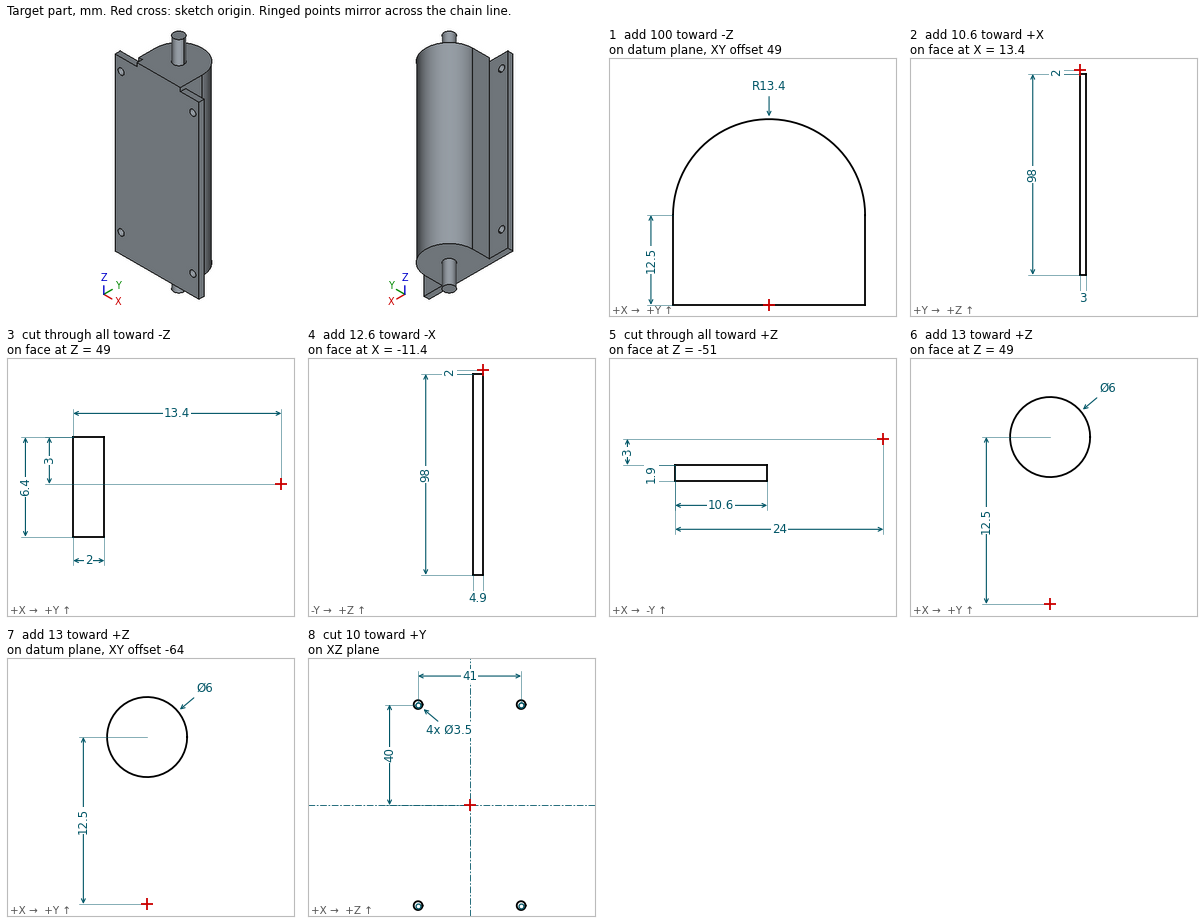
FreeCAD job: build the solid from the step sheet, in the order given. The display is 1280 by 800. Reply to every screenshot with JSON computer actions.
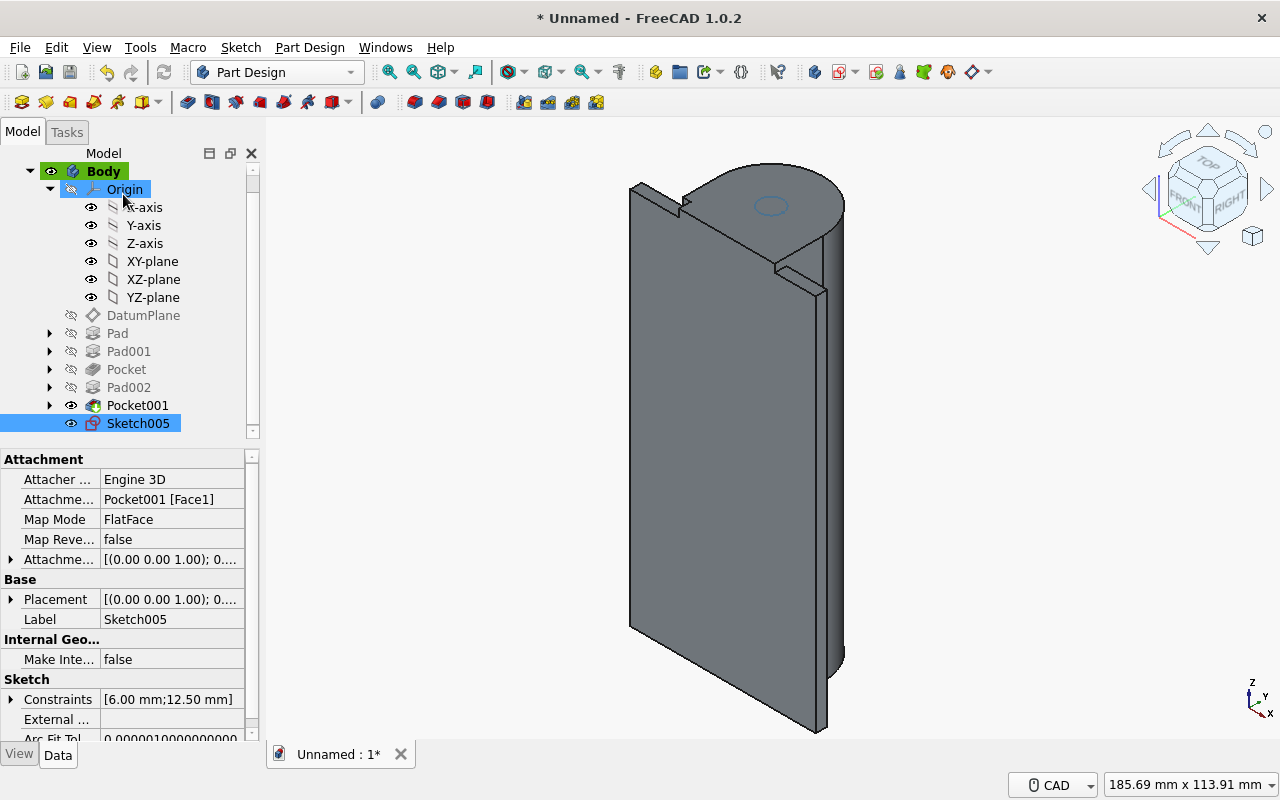
{"action": "left_click", "coordinate": [22, 102]}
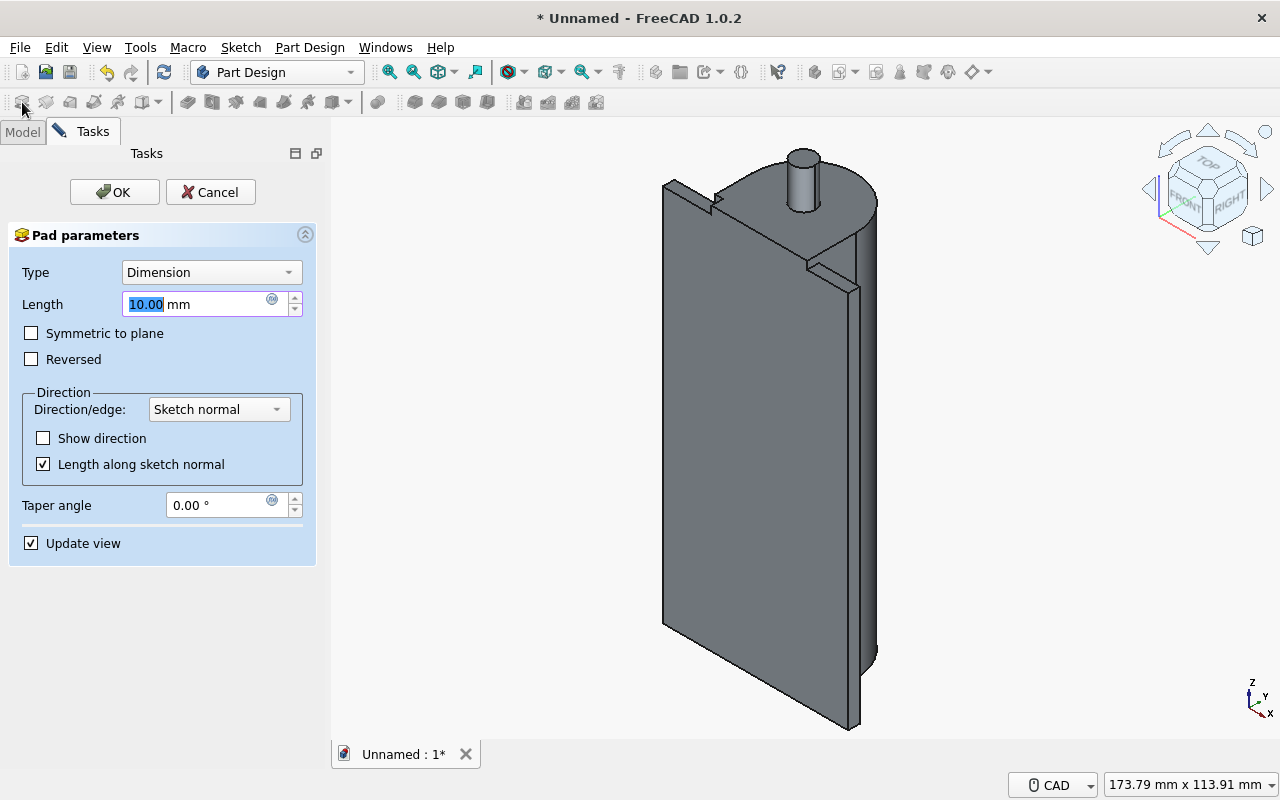
{"action": "type", "text": "13"}
{"action": "key", "text": "Tab"}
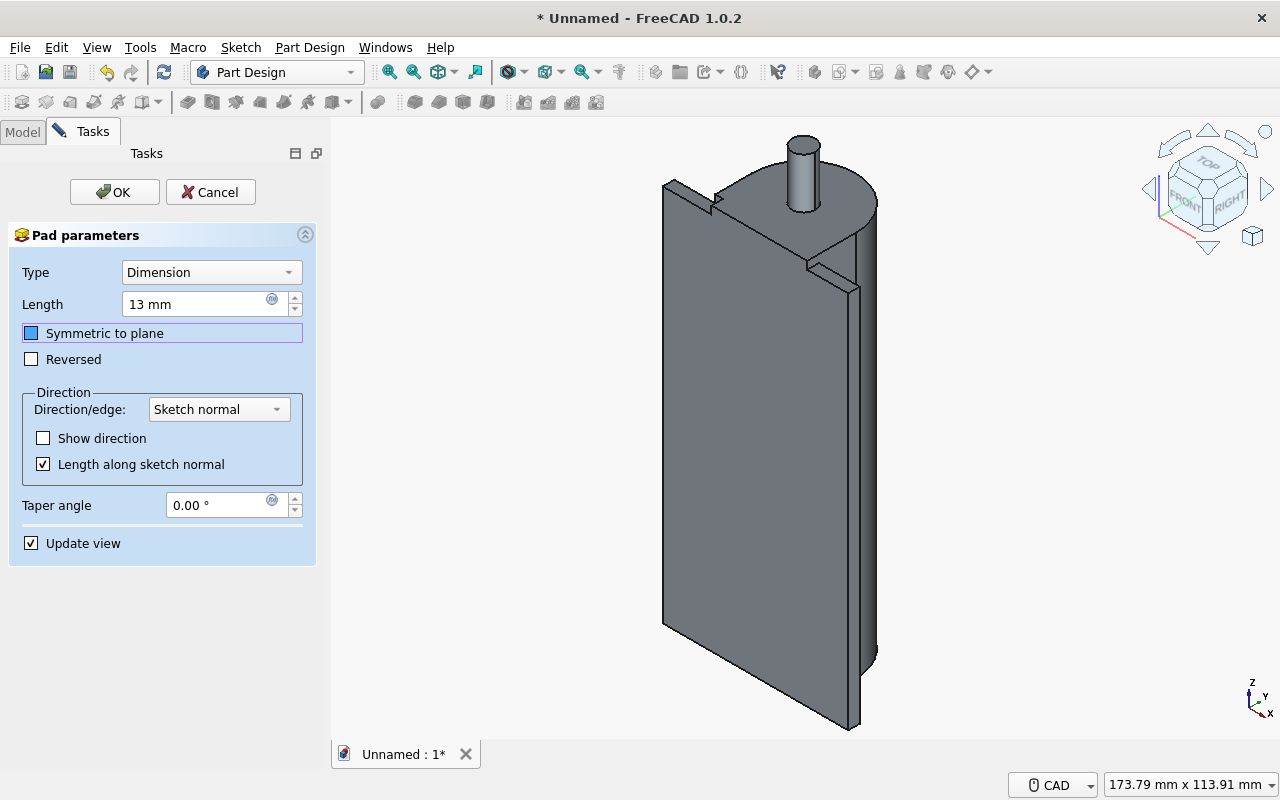
{"action": "left_click", "coordinate": [115, 192]}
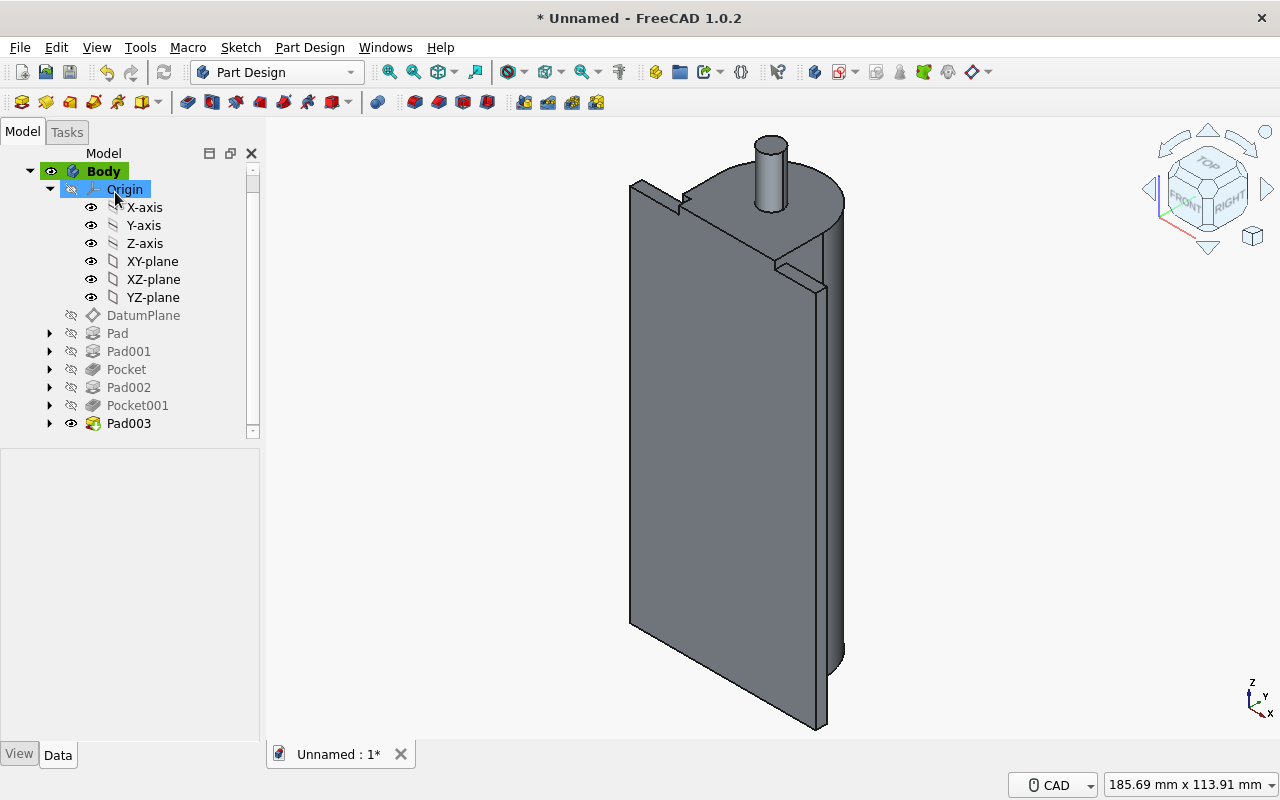
{"action": "left_click", "coordinate": [390, 72]}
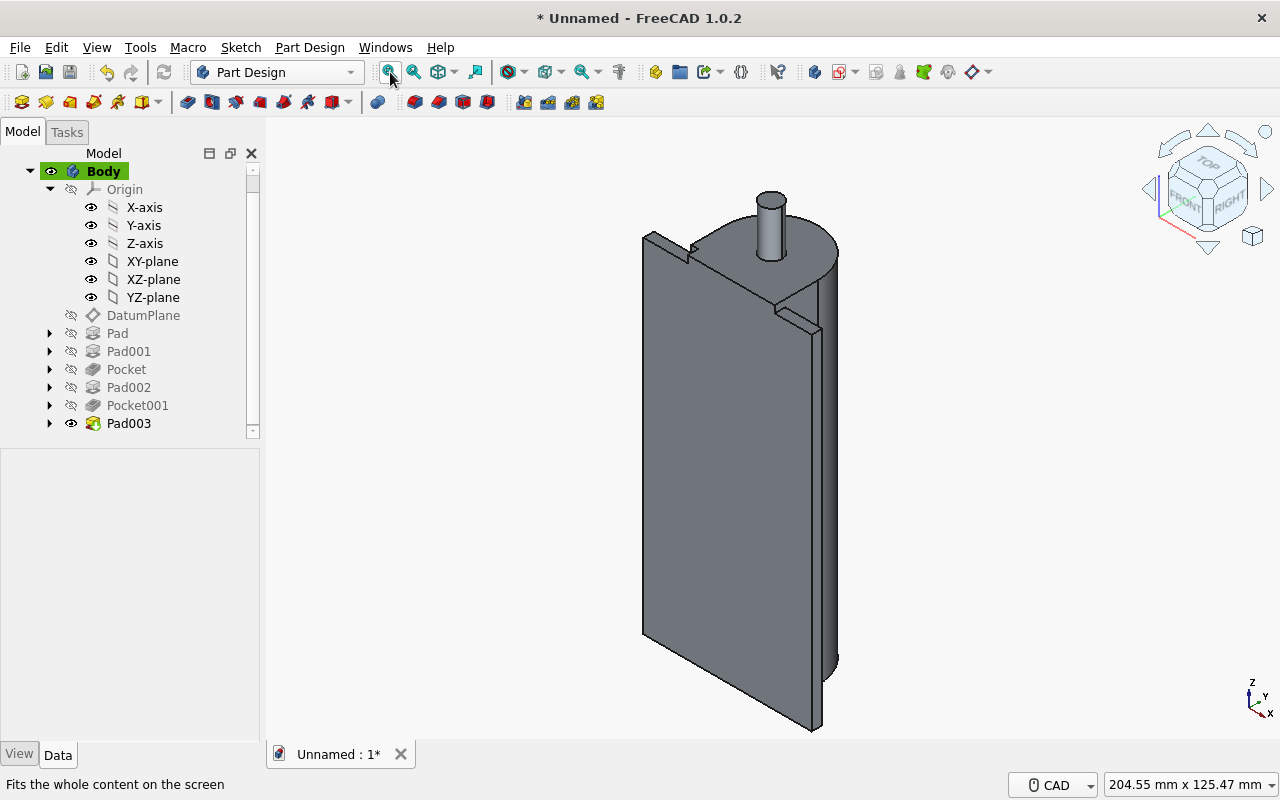
{"action": "left_click", "coordinate": [136, 261]}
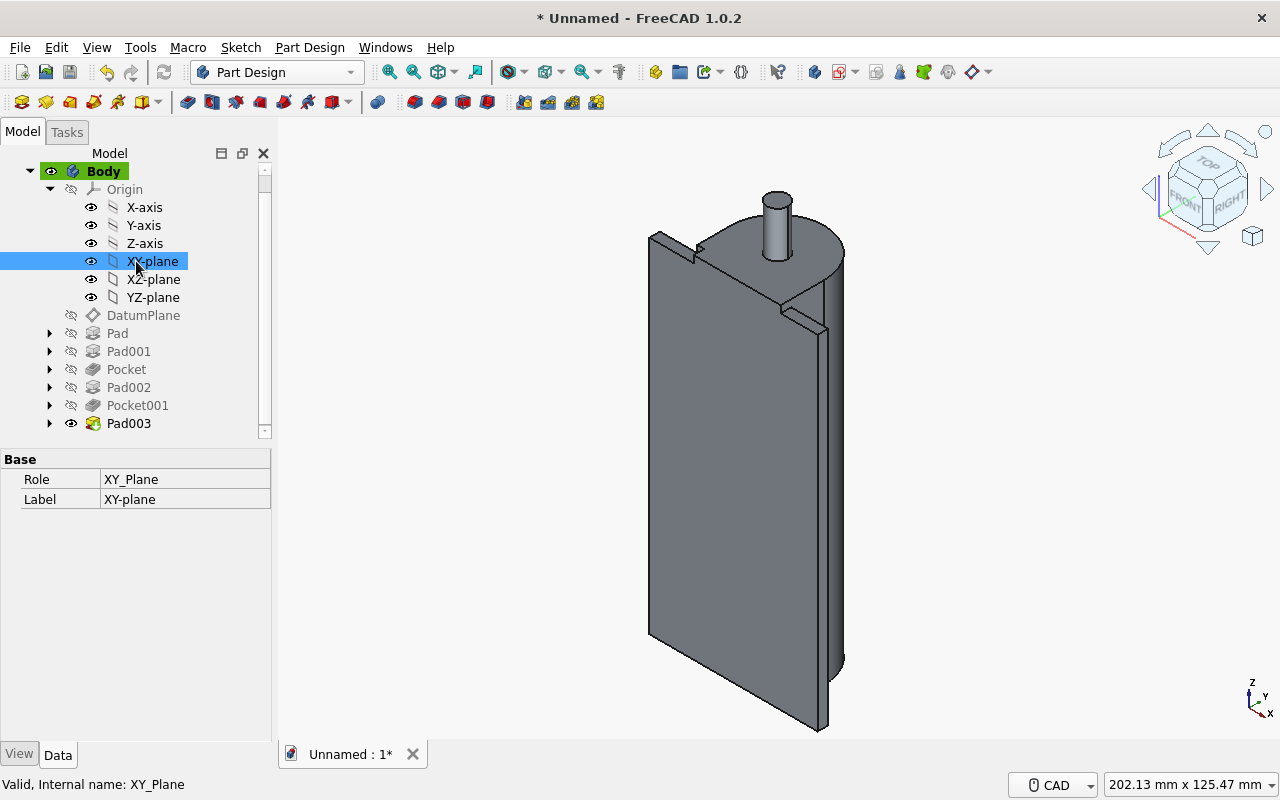
{"action": "left_click", "coordinate": [972, 72]}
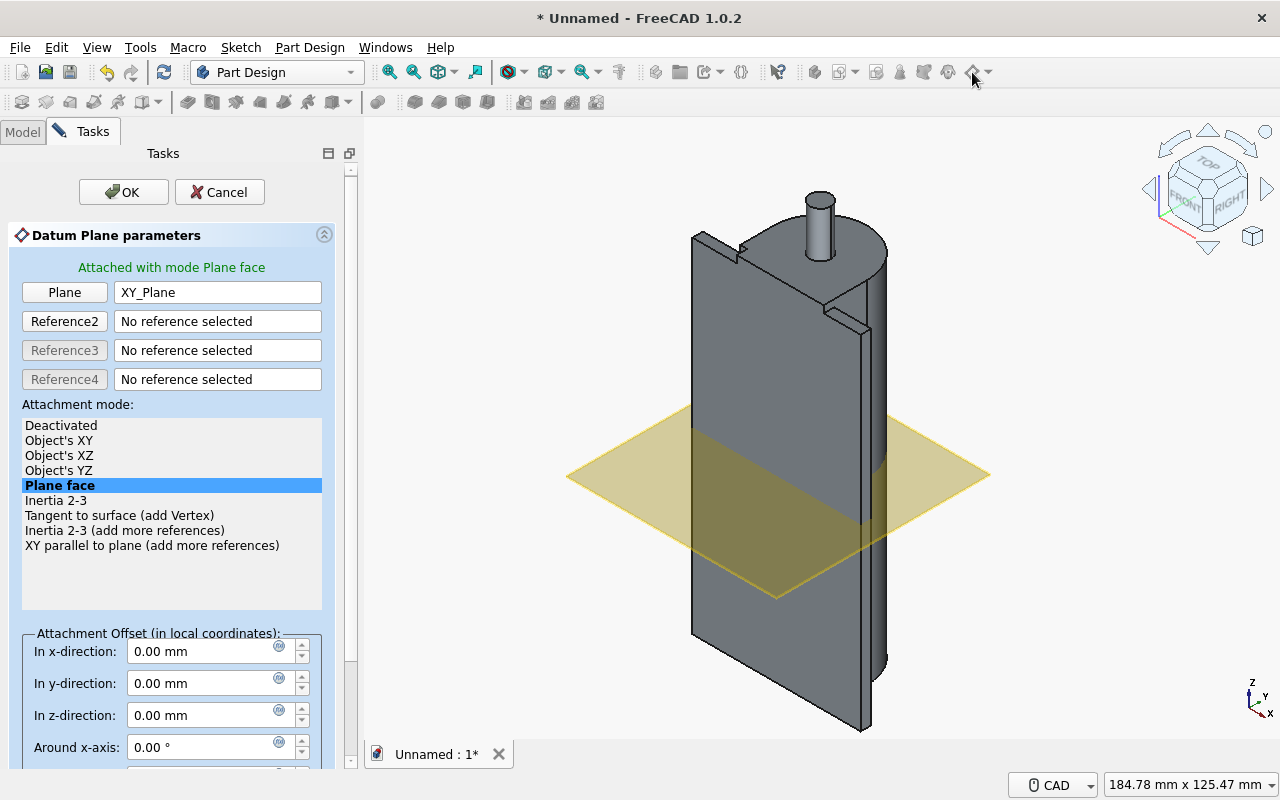
{"action": "triple_click", "coordinate": [210, 715]}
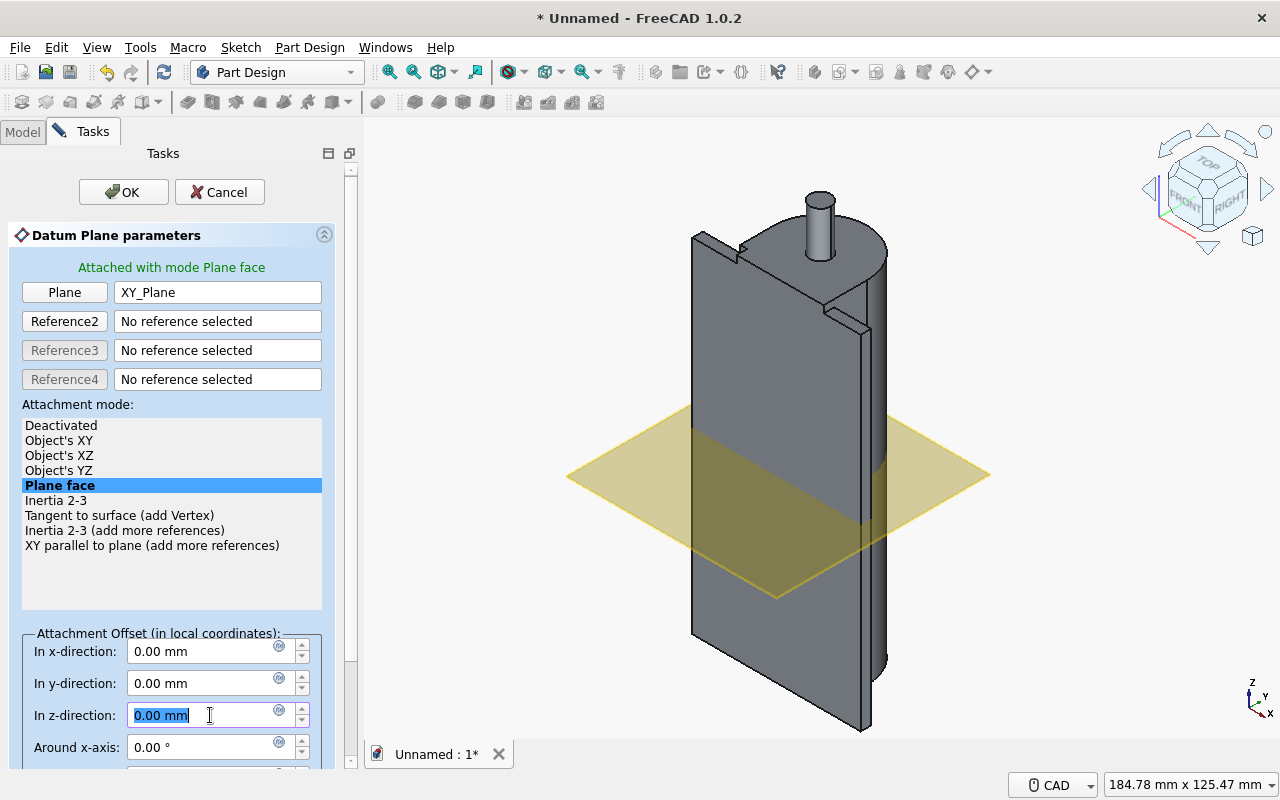
{"action": "type", "text": "-64"}
{"action": "key", "text": "Tab"}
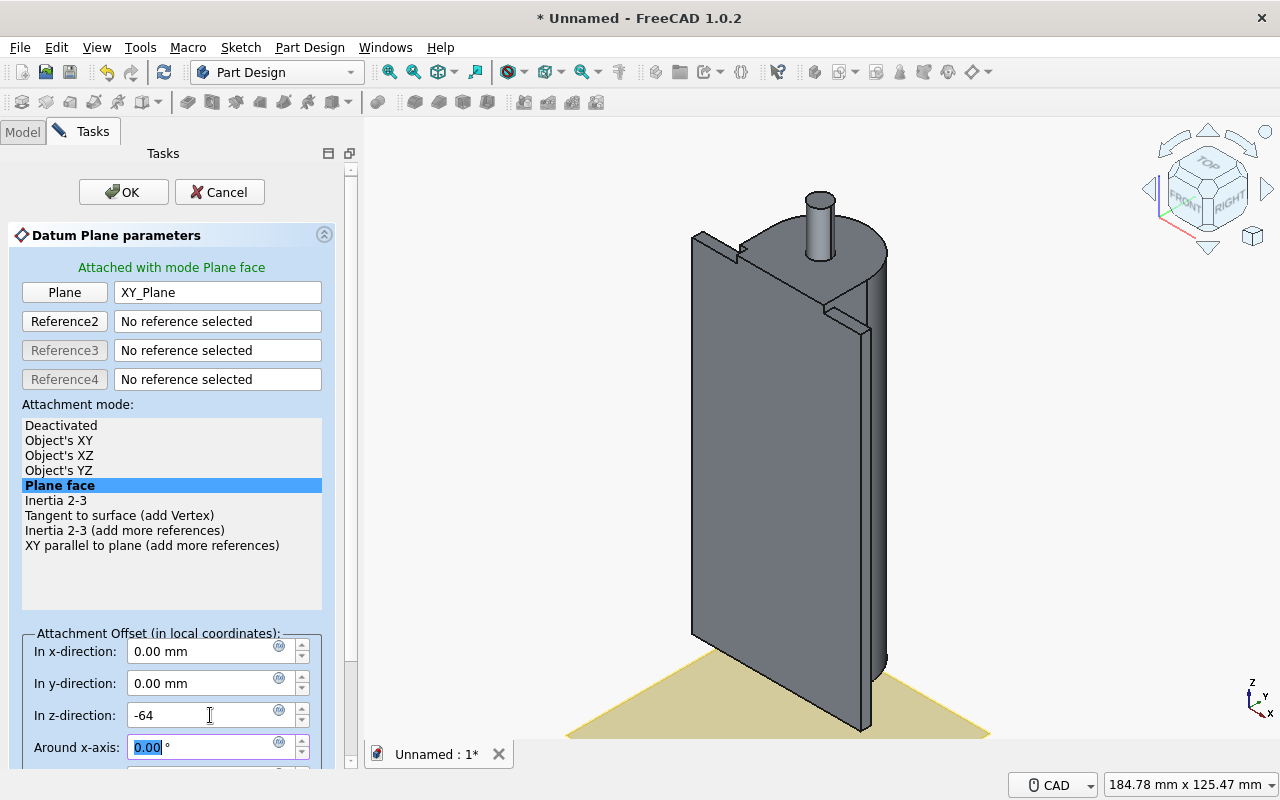
{"action": "left_click", "coordinate": [124, 192]}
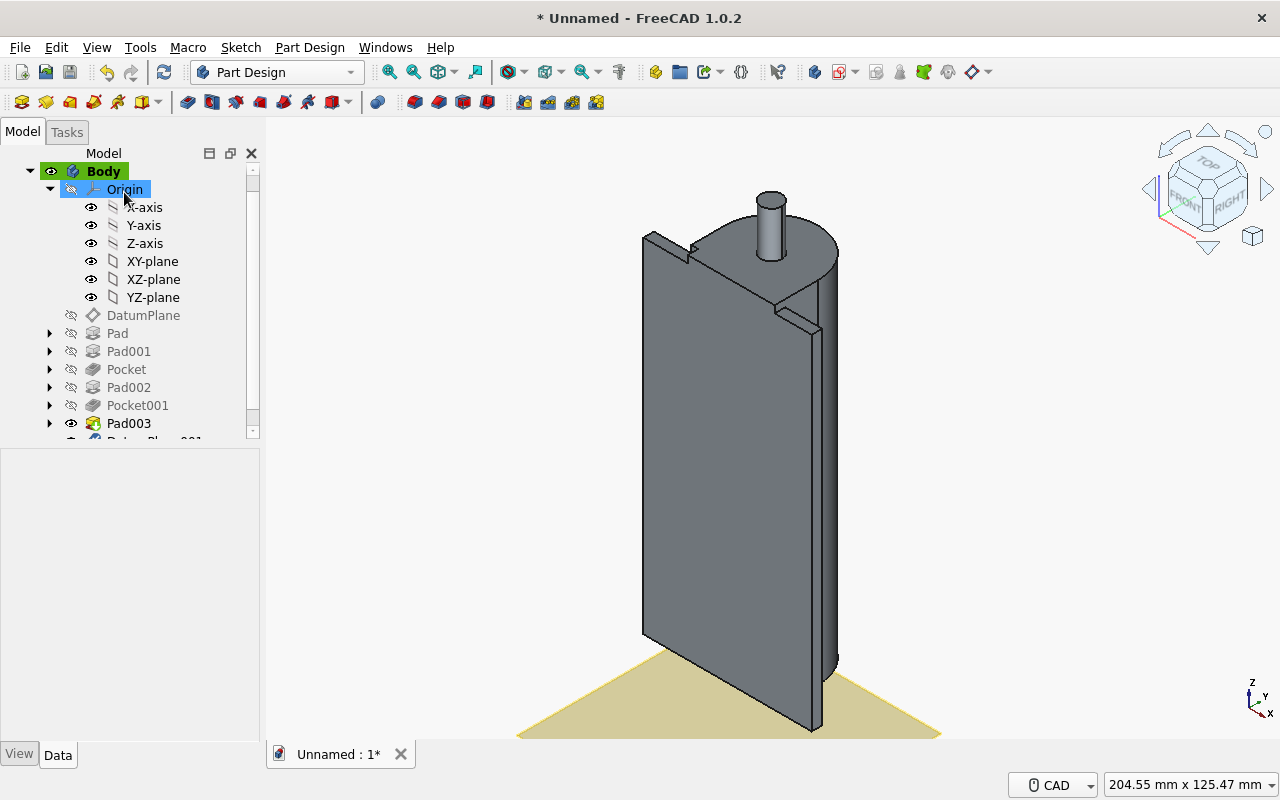
{"action": "scroll", "coordinate": [120, 293], "scroll_direction": "down", "scroll_amount": 3}